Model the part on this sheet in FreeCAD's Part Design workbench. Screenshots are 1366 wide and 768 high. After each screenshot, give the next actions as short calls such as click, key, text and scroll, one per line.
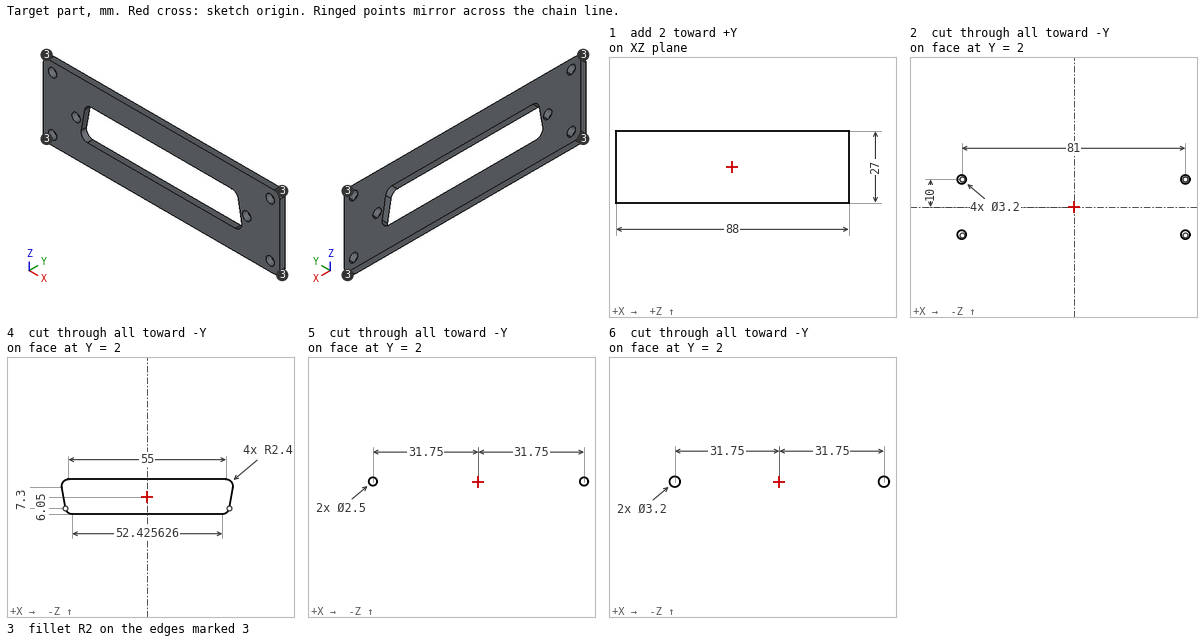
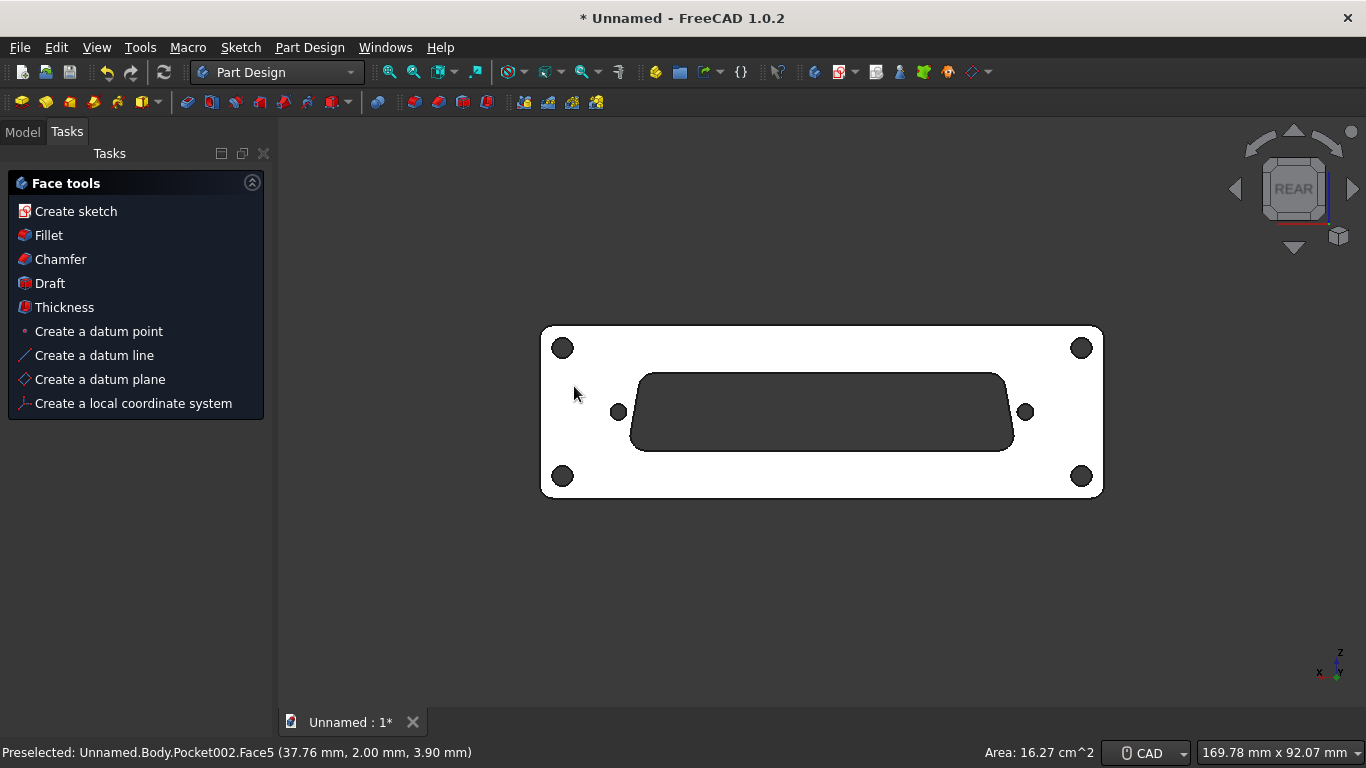
click(840, 72)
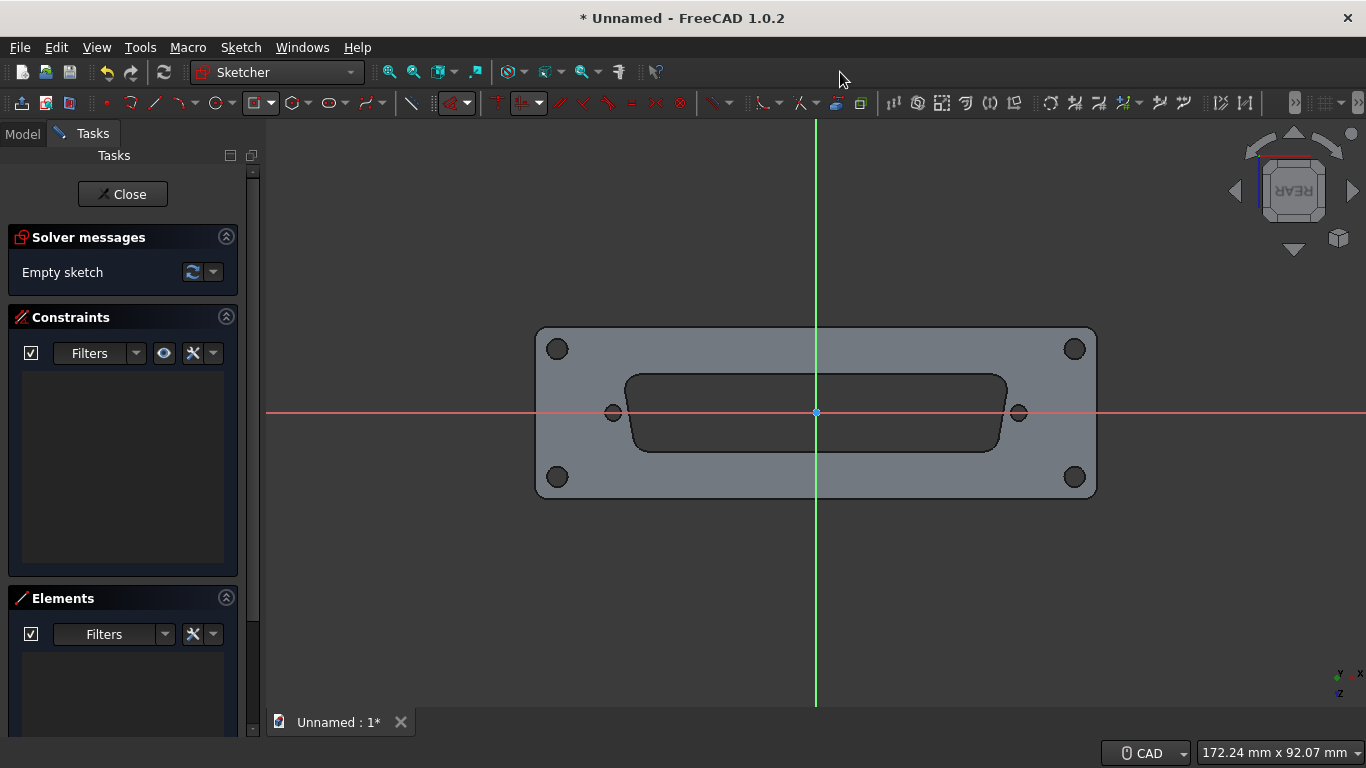
scroll(955, 413, up, 2)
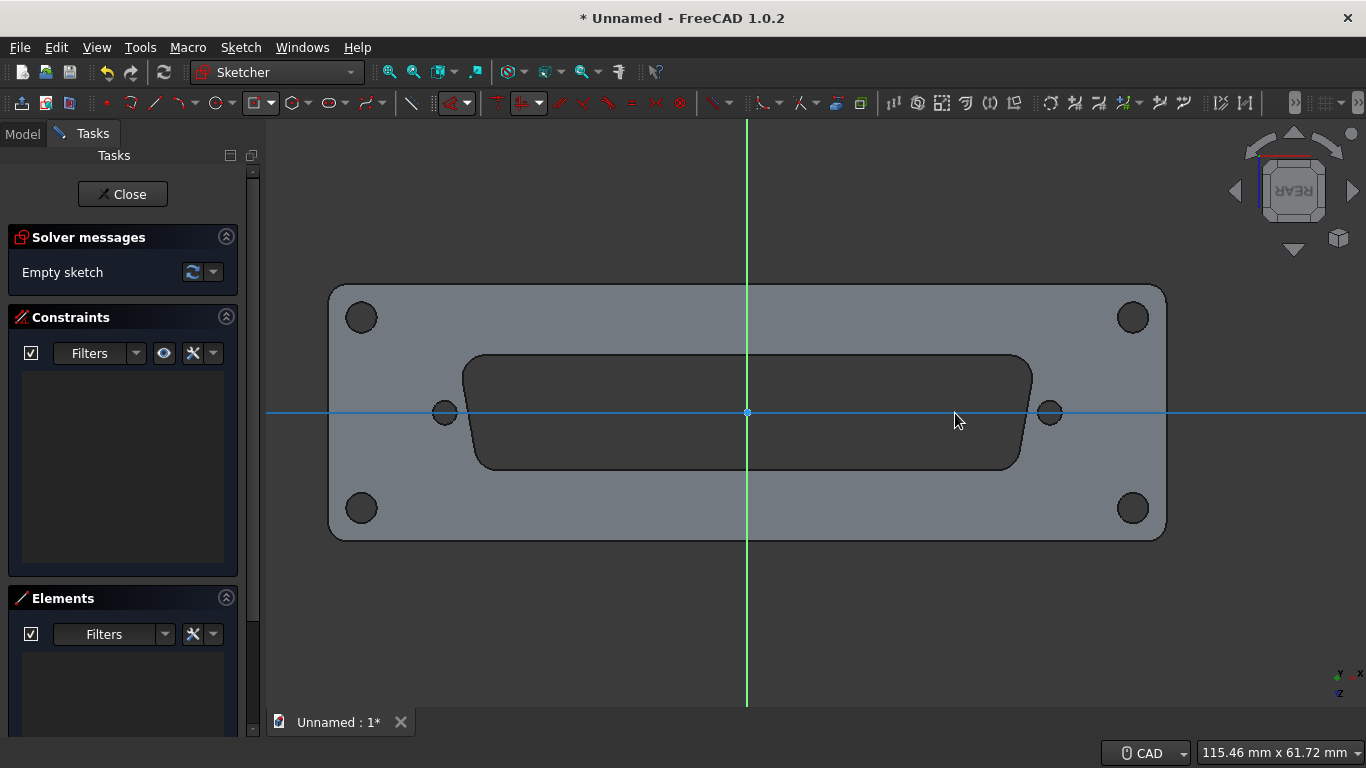
key(g)
key(c)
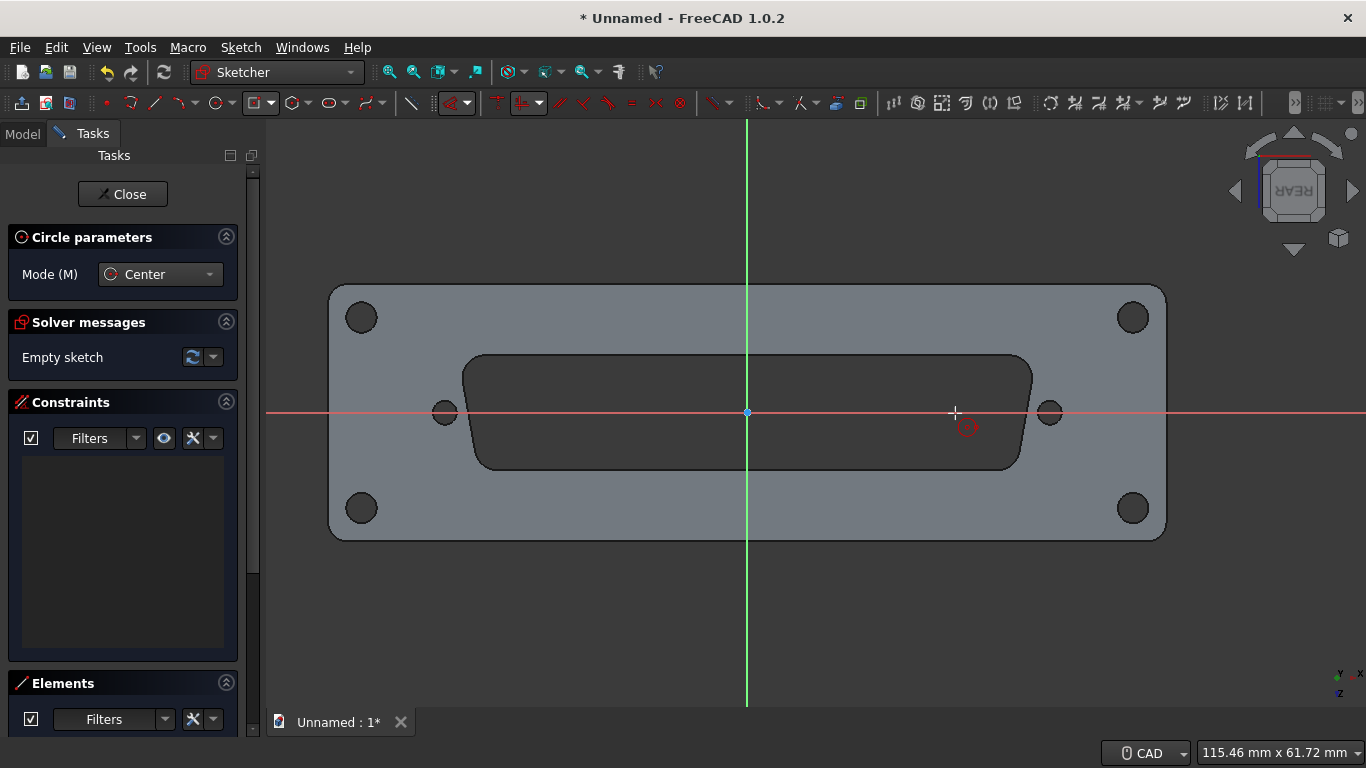
scroll(445, 413, up, 2)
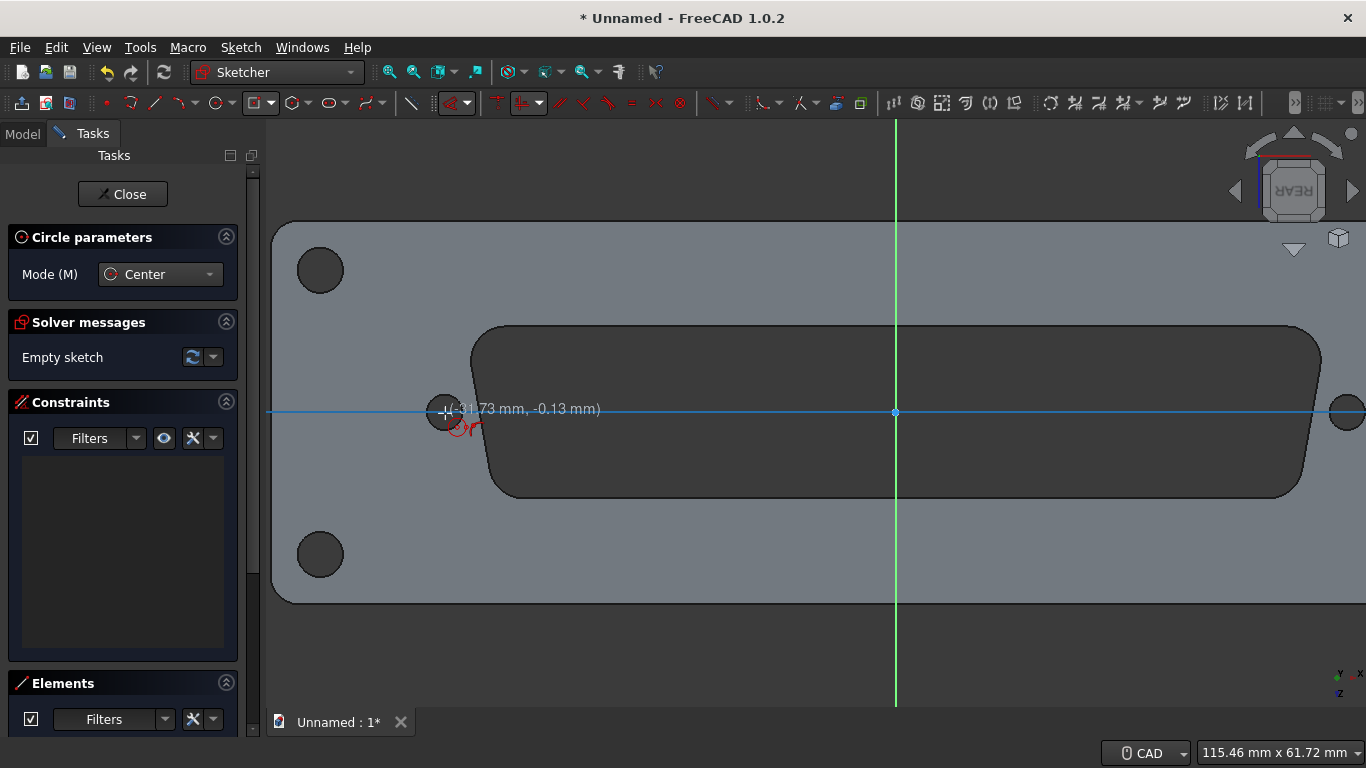
click(445, 412)
click(461, 396)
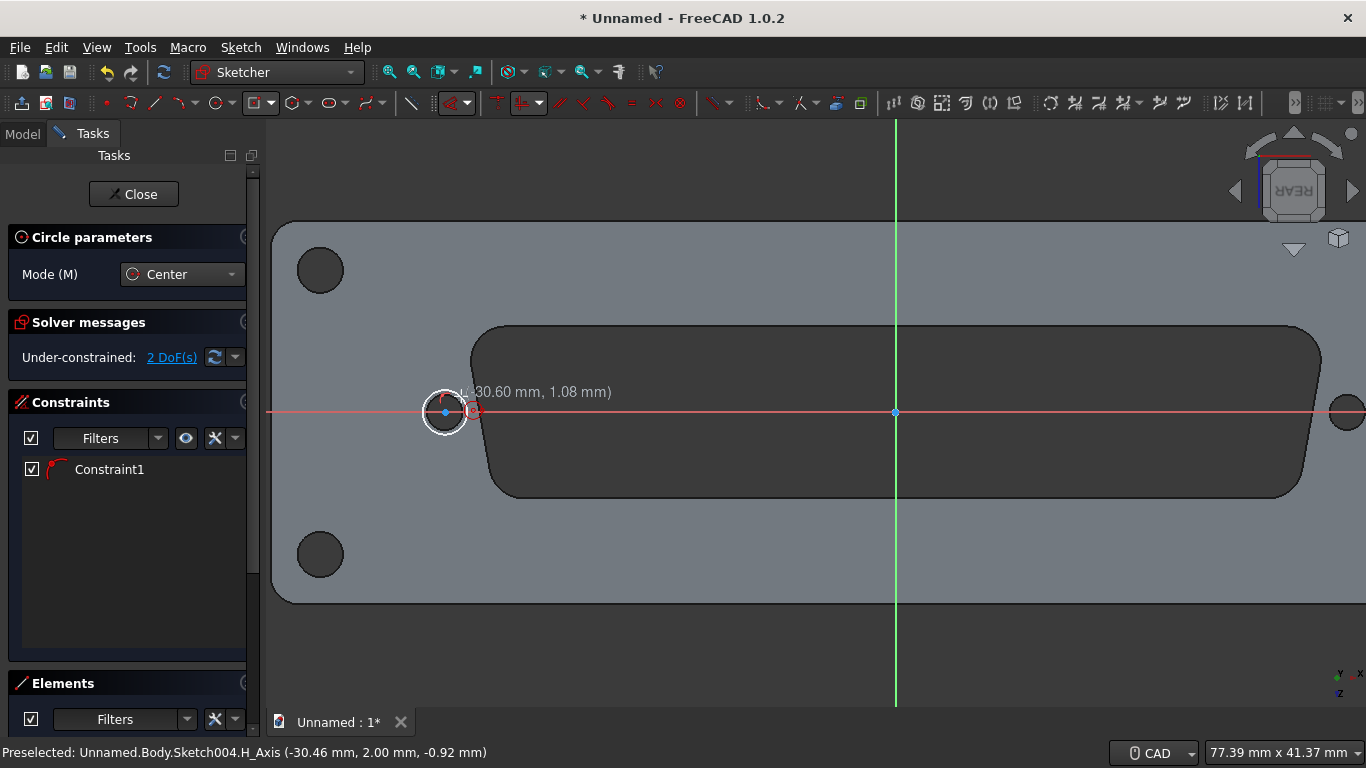
scroll(446, 414, down, 2)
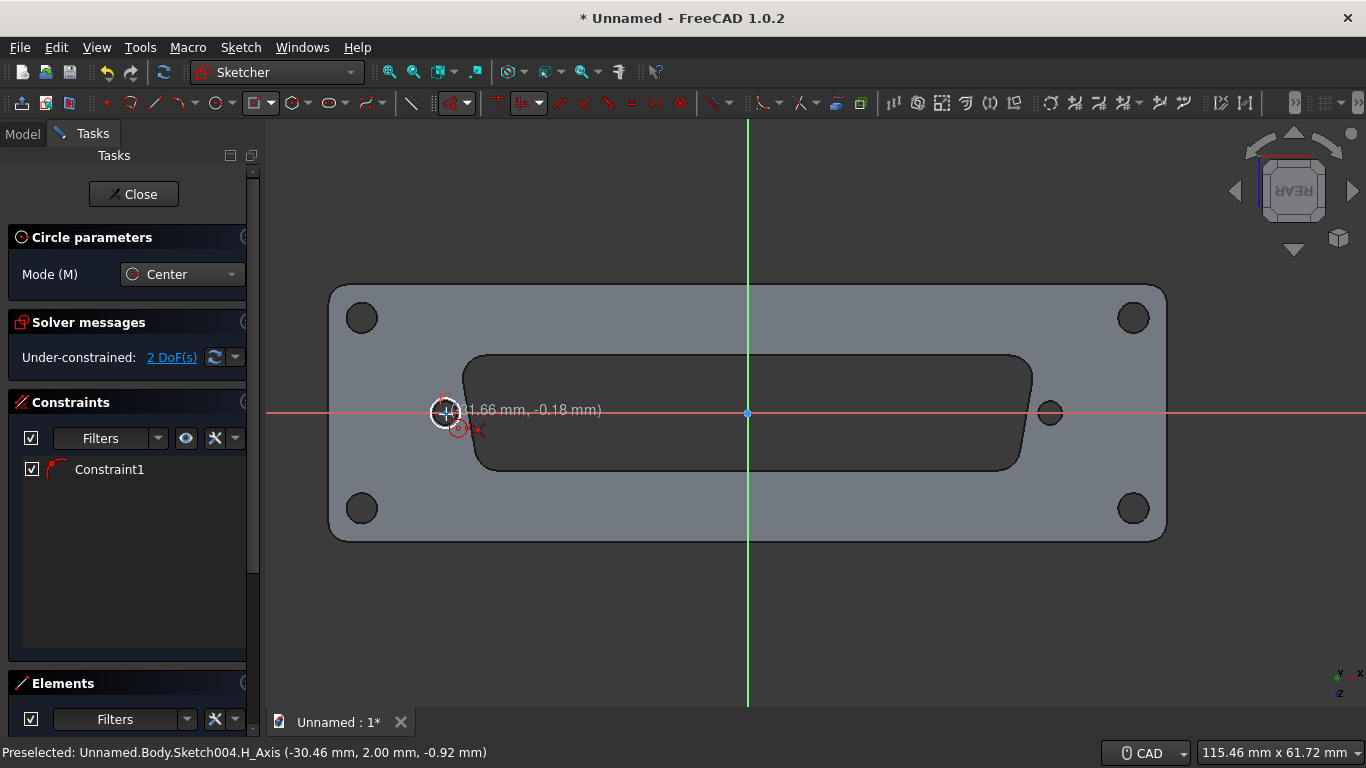
scroll(1050, 413, up, 2)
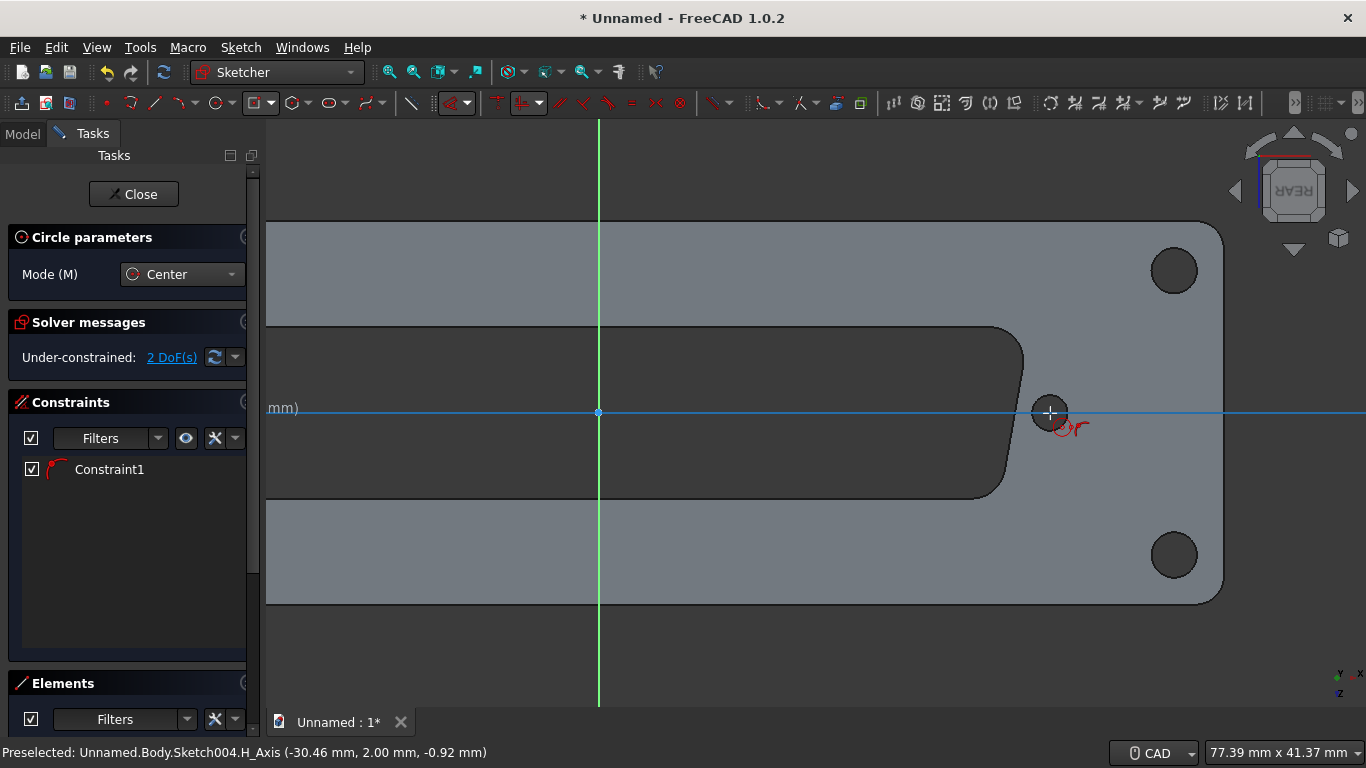
click(1050, 413)
click(1066, 397)
key(Escape)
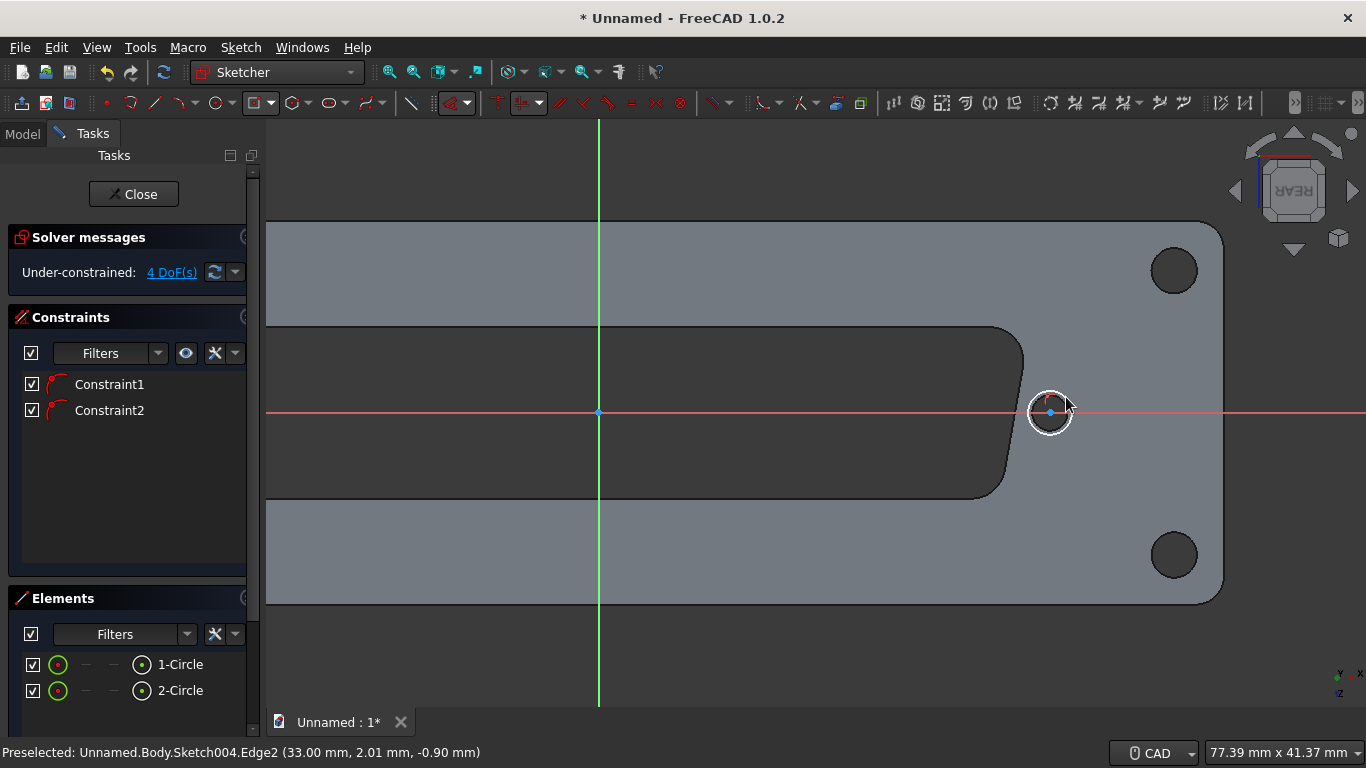
scroll(1050, 413, down, 2)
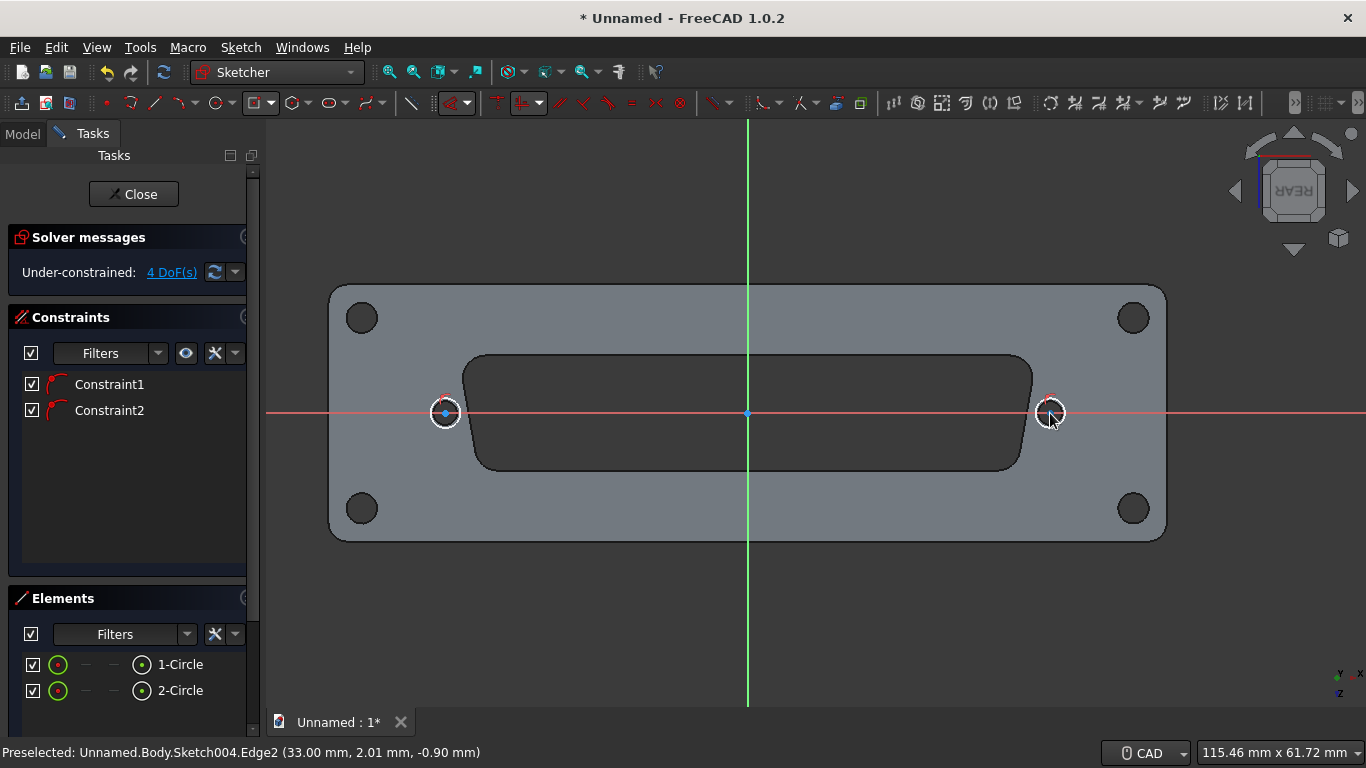
scroll(456, 403, up, 2)